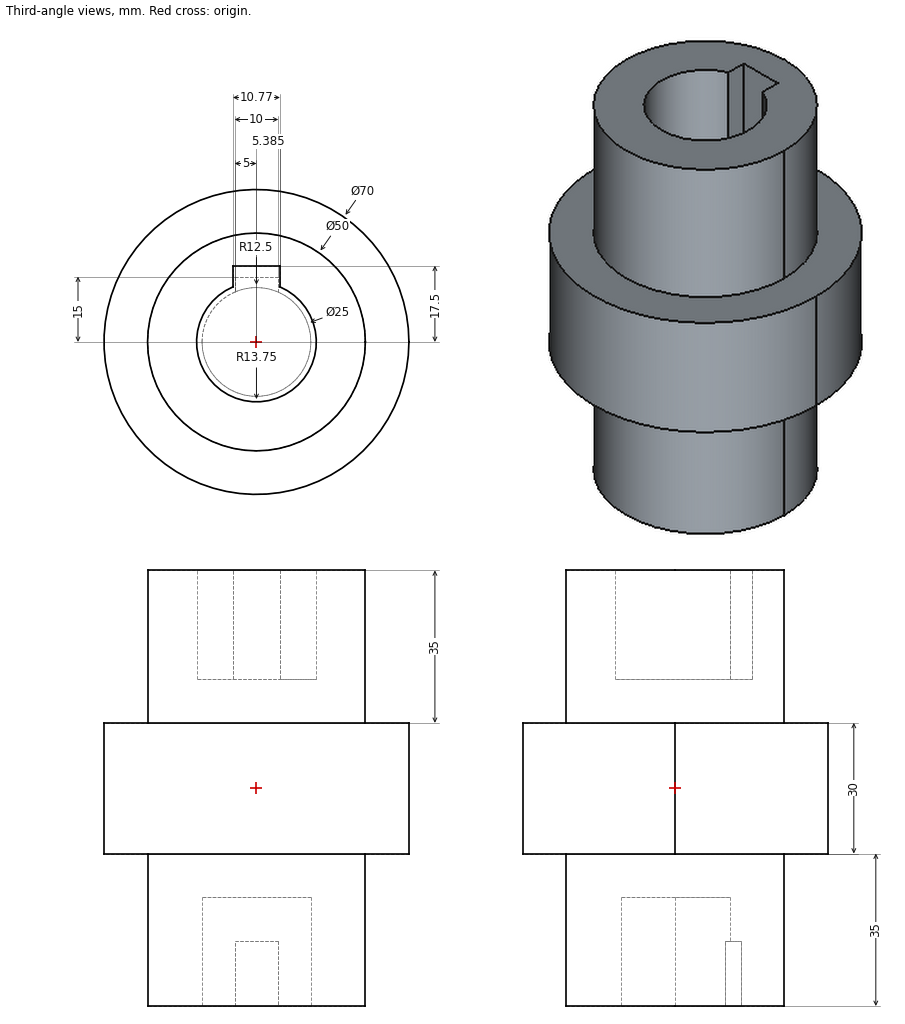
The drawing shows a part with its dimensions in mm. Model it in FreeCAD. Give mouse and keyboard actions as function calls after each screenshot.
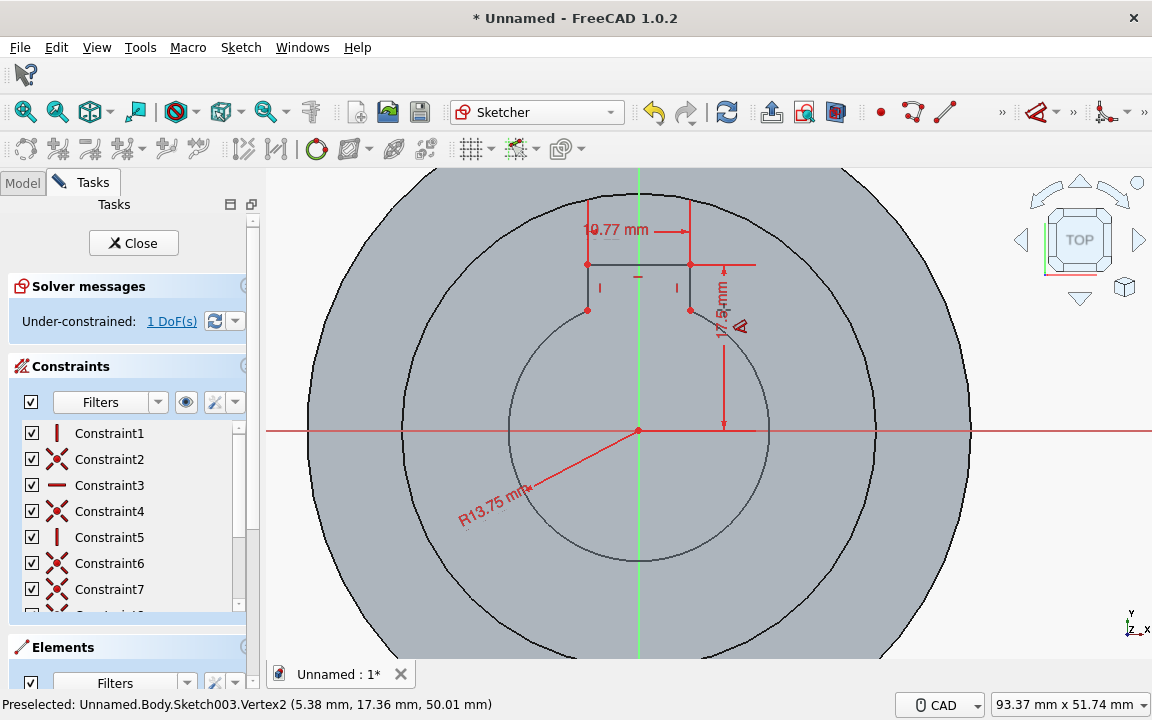
click(690, 311)
click(664, 465)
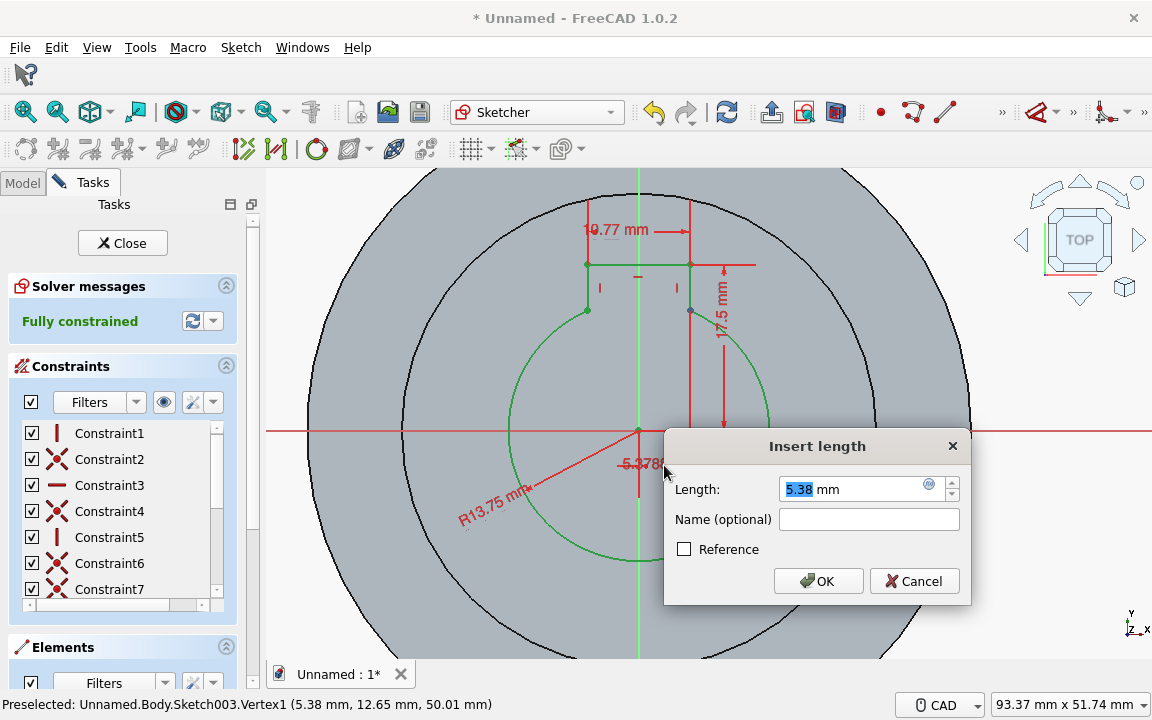
text(5.385)
key(Return)
key(Escape)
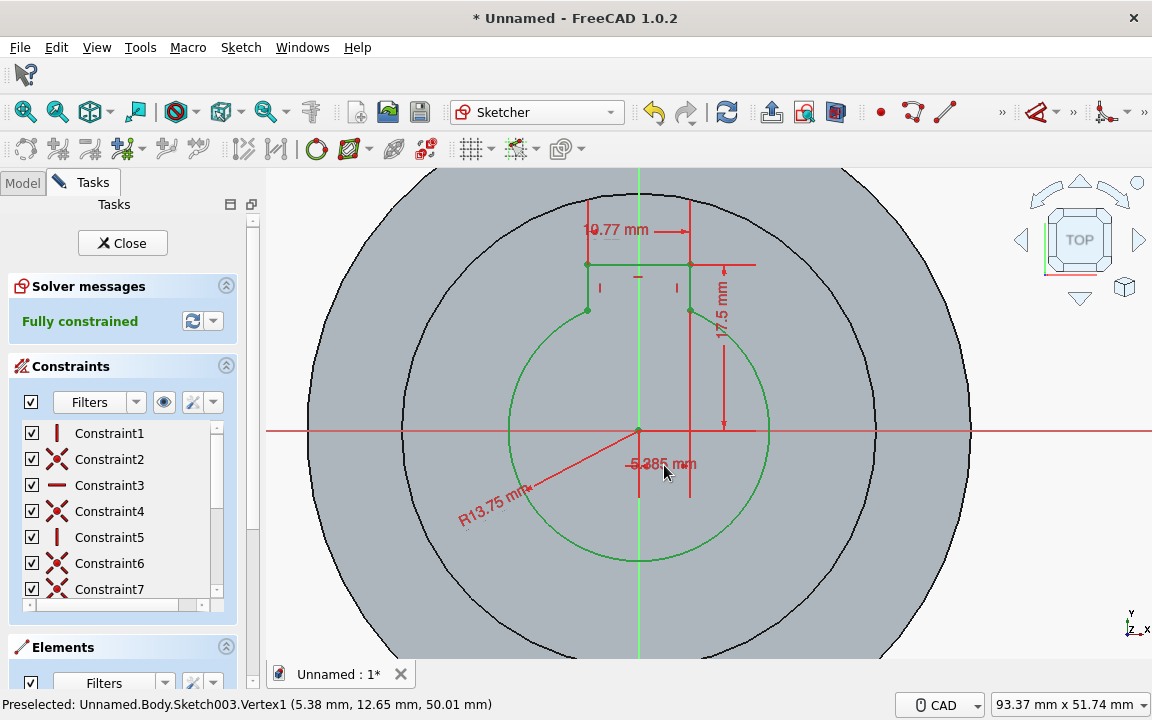
click(123, 243)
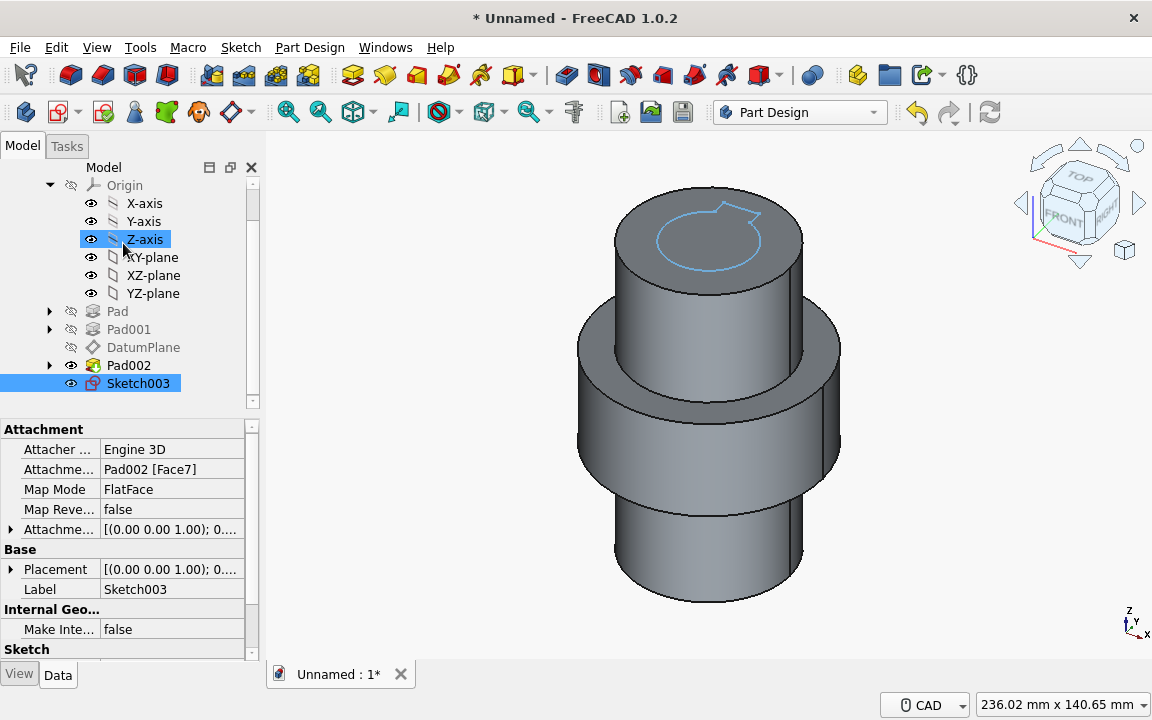
click(568, 76)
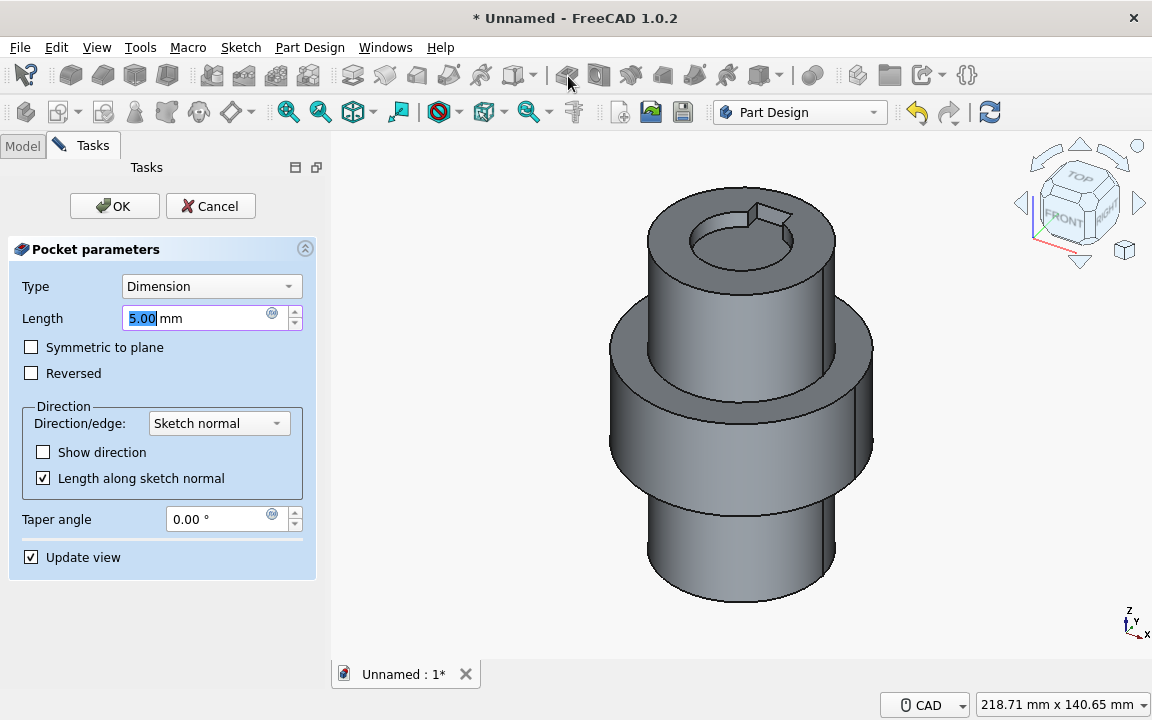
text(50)
key(Tab)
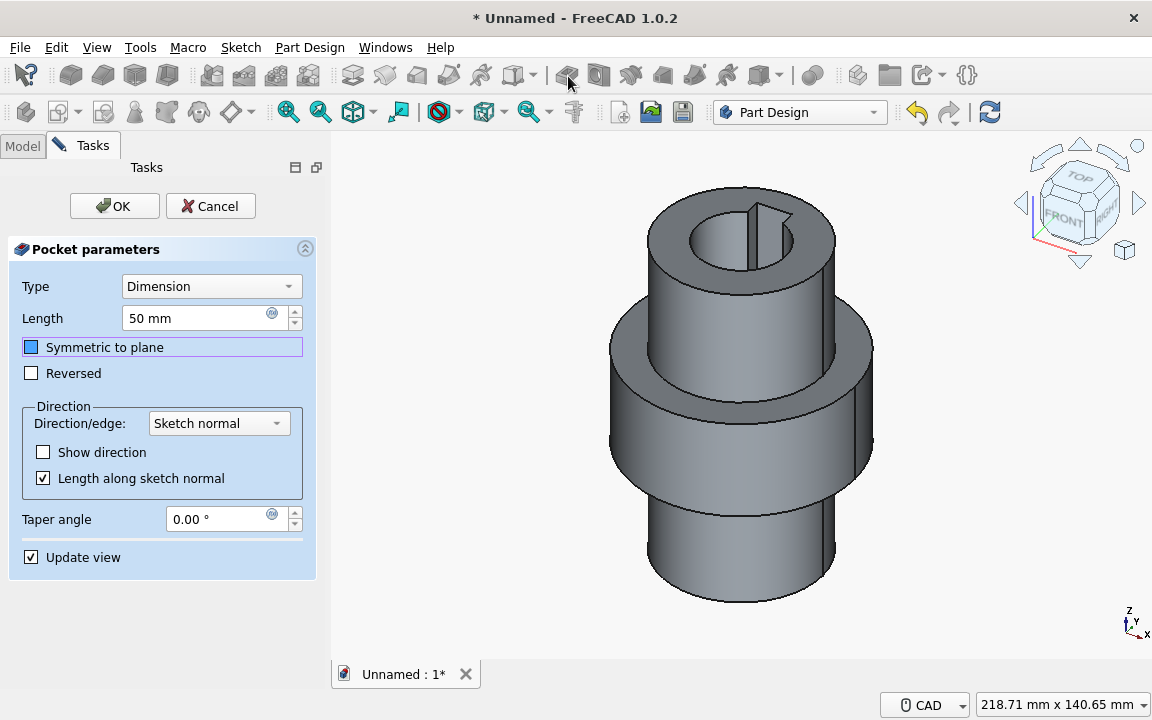
click(30, 347)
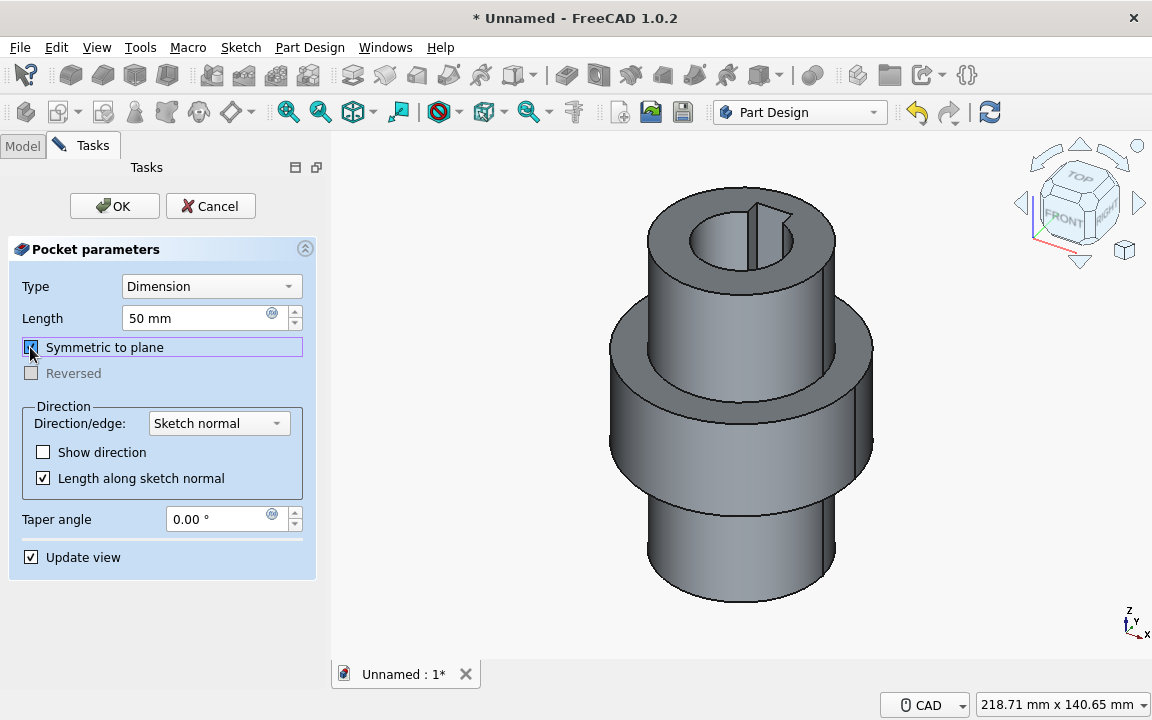
click(115, 206)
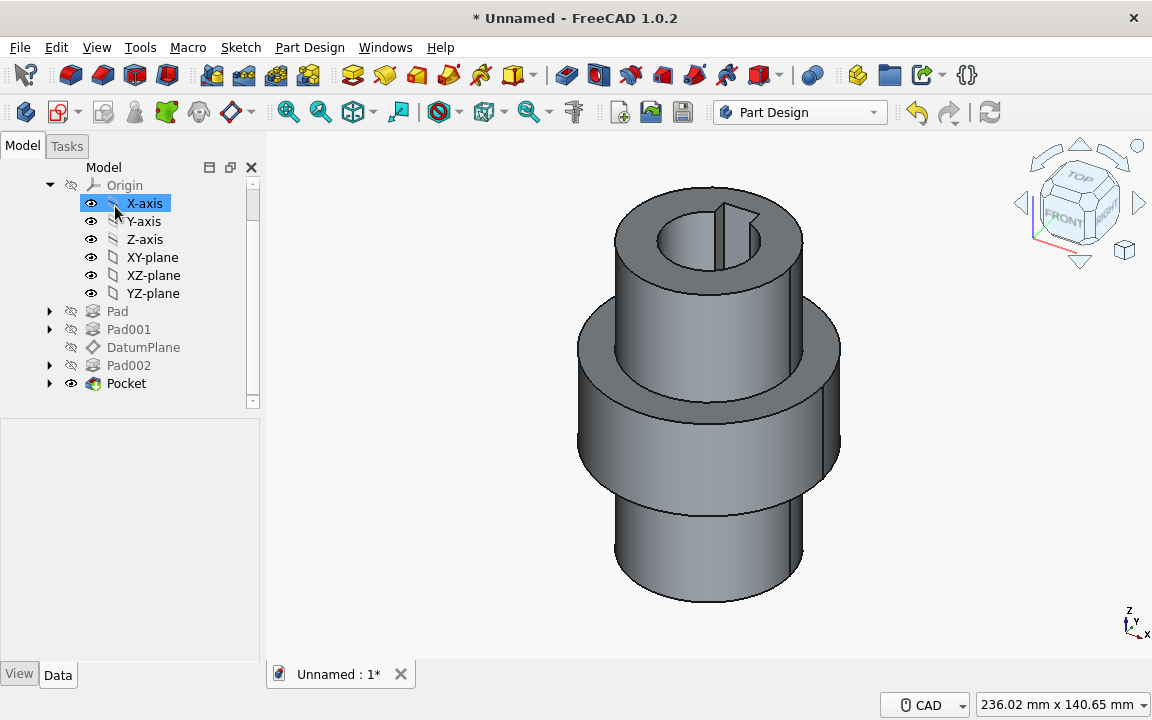
key(5)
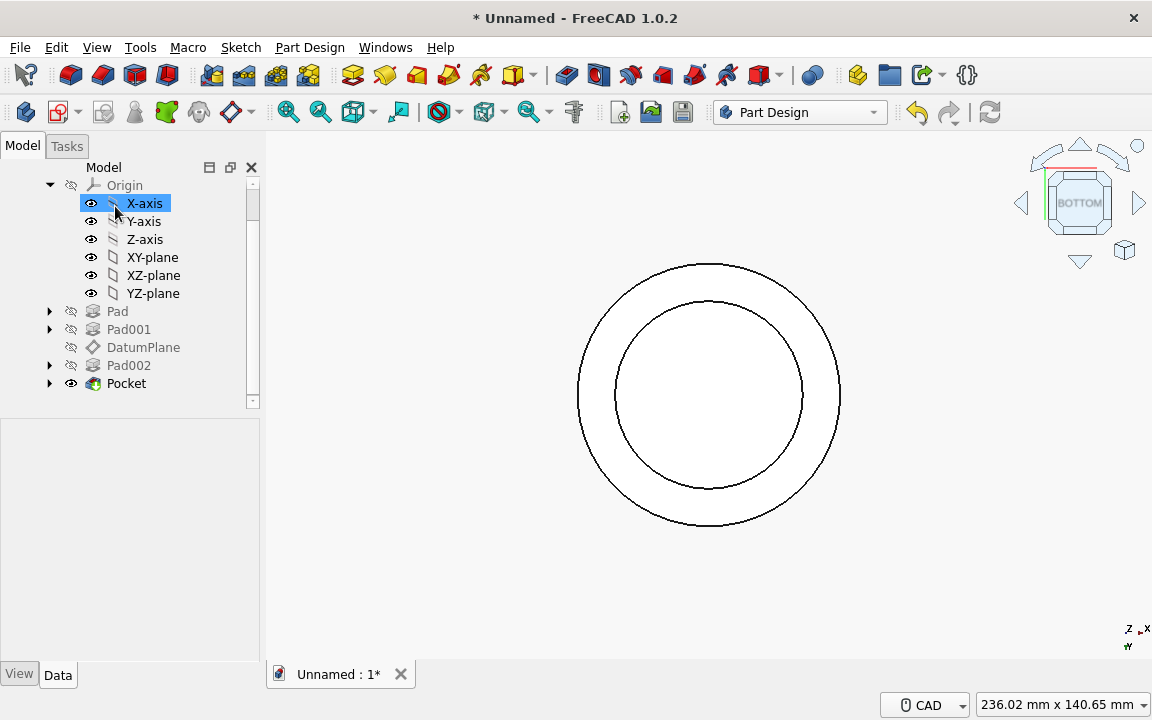
click(709, 394)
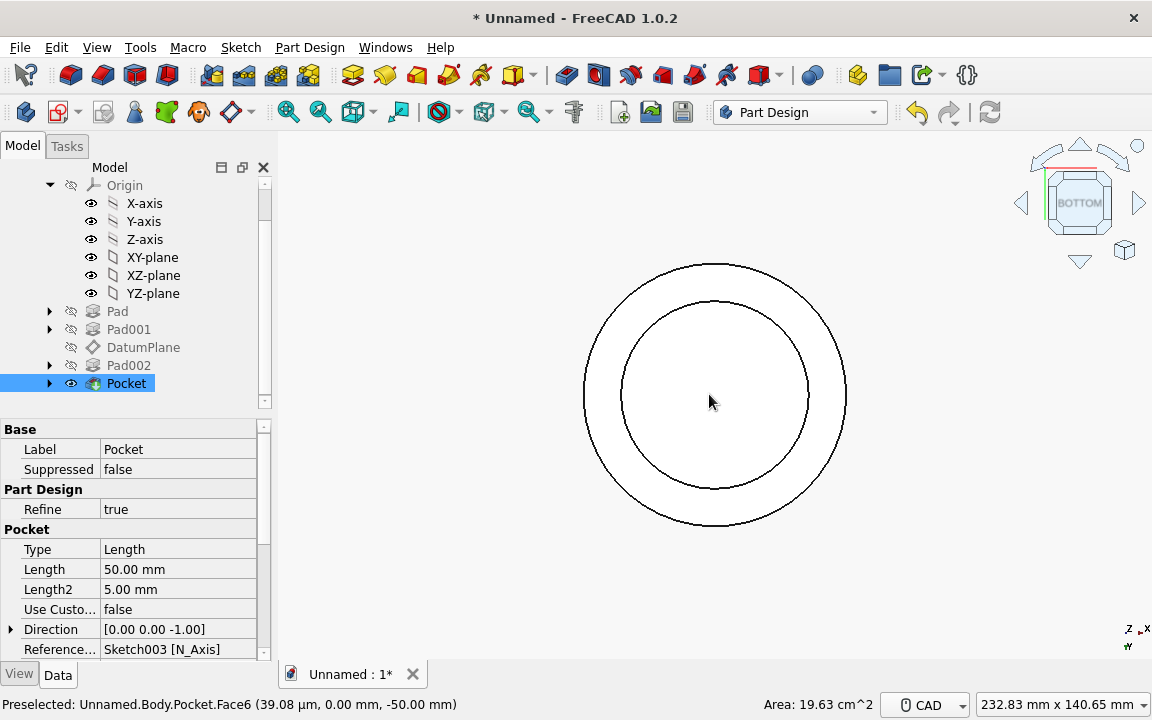
click(58, 112)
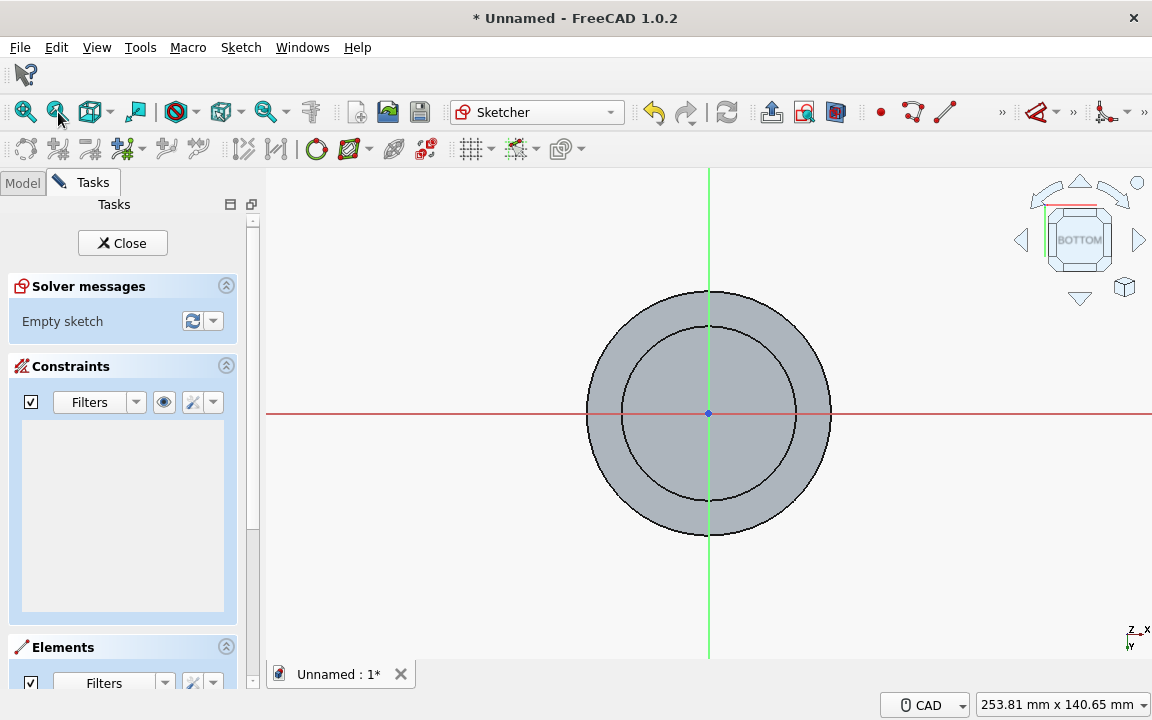
scroll(738, 414, up, 6)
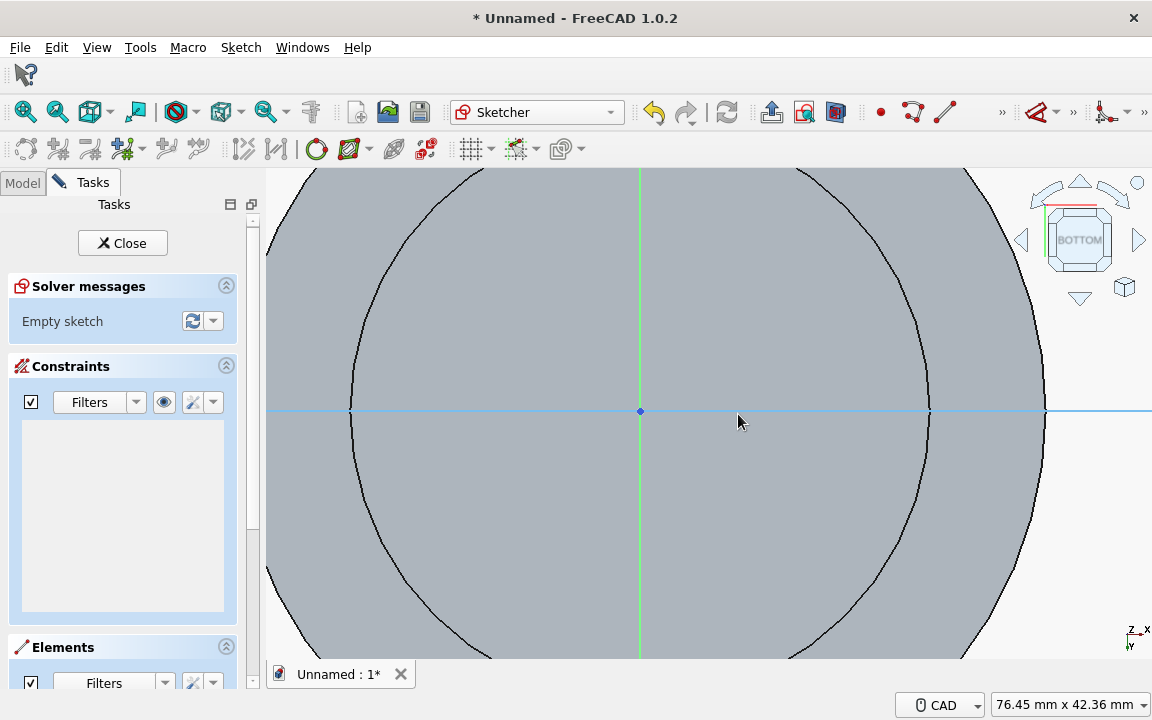
key(g)
key(c)